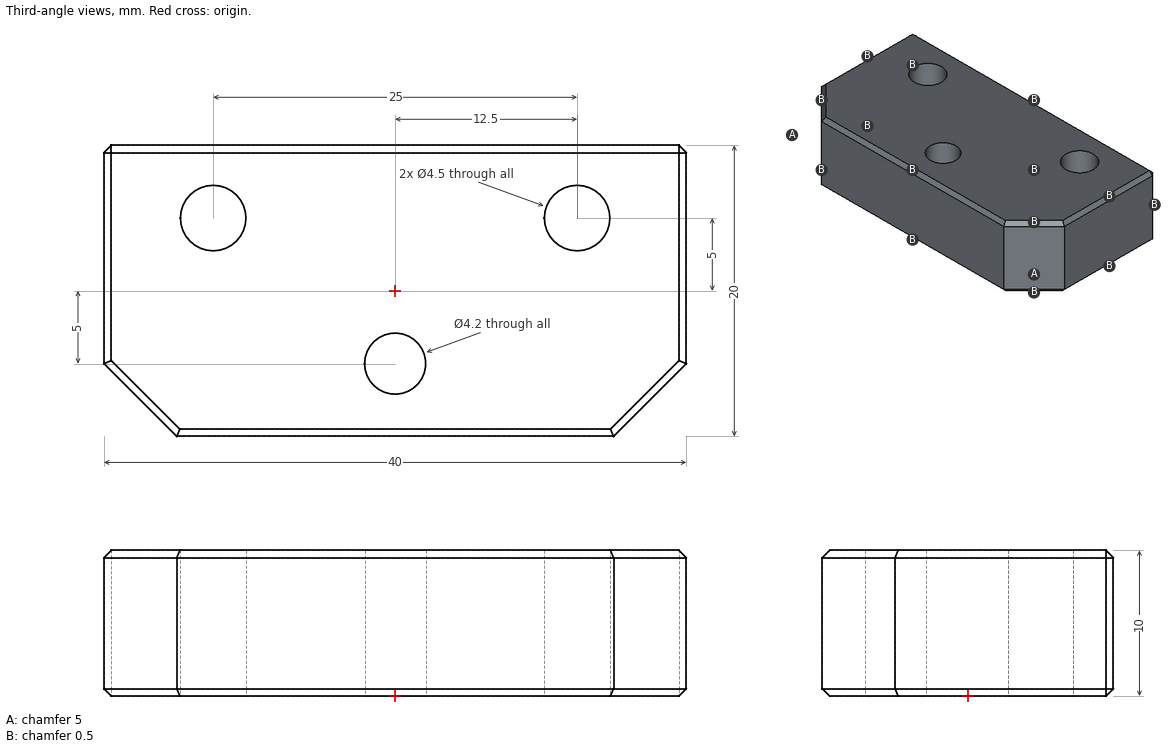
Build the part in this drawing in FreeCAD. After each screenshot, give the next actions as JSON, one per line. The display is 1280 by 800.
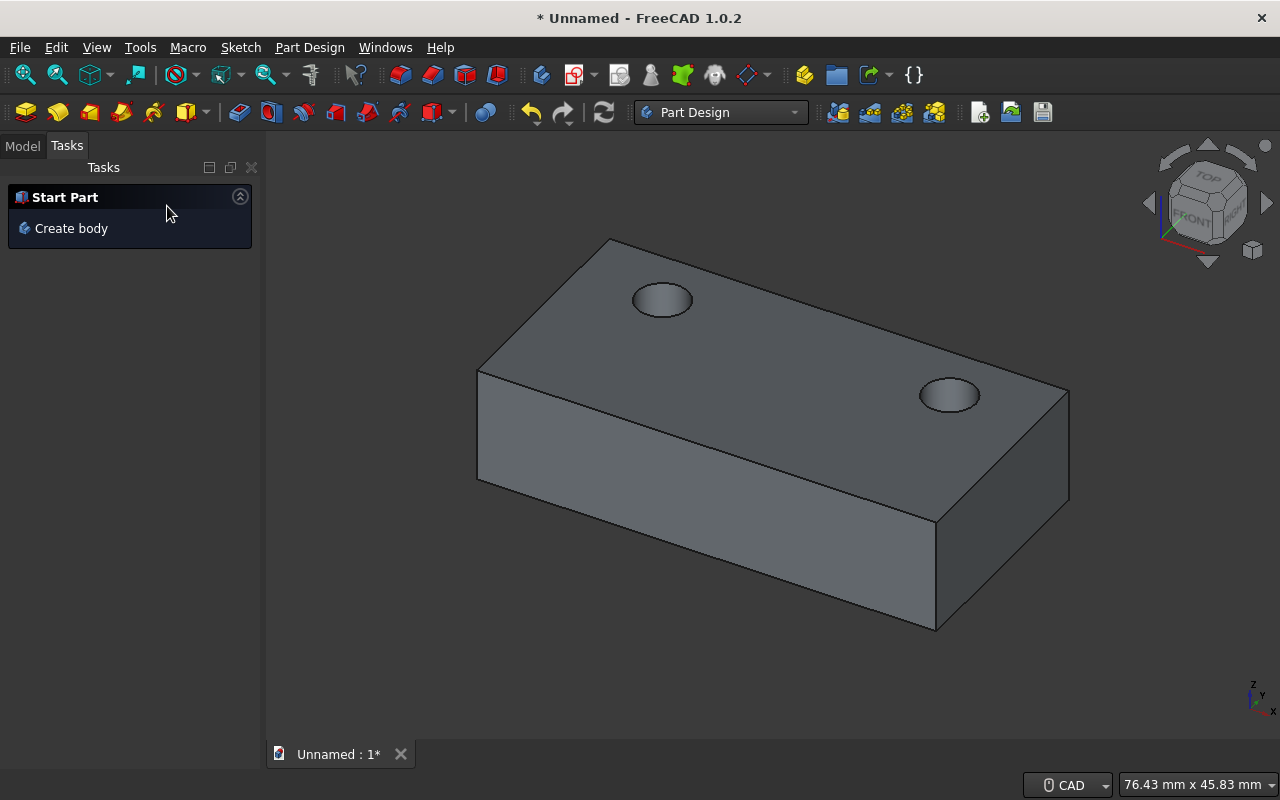
{"action": "left_click", "coordinate": [773, 380]}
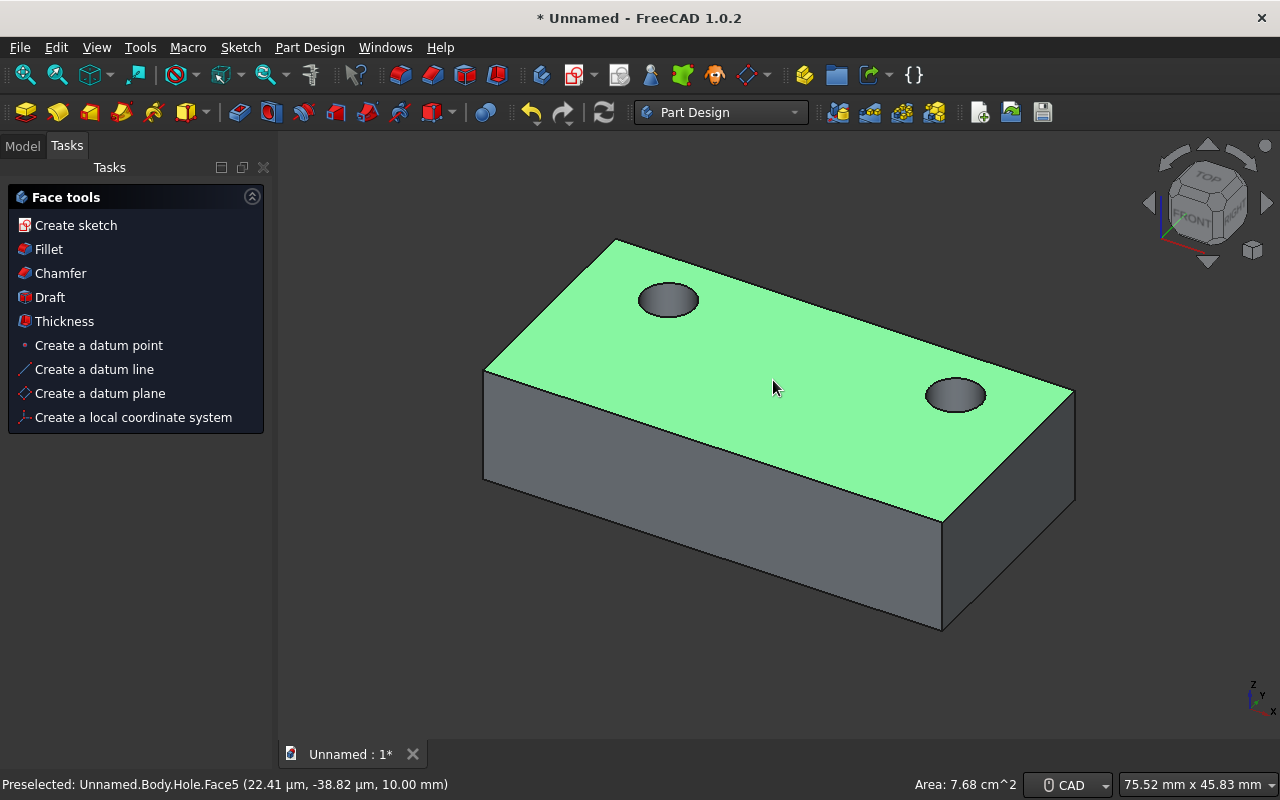
{"action": "left_click", "coordinate": [574, 76]}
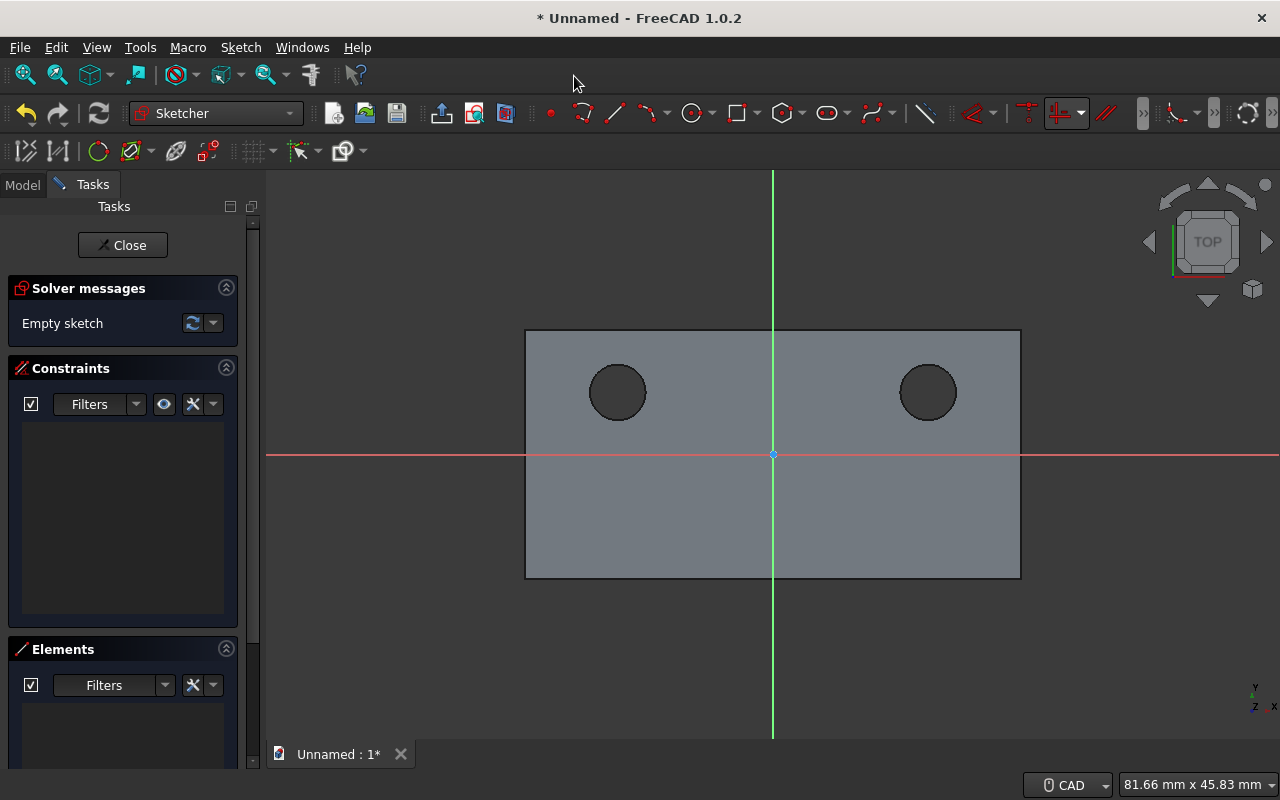
{"action": "scroll", "coordinate": [795, 513], "scroll_direction": "up", "scroll_amount": 7}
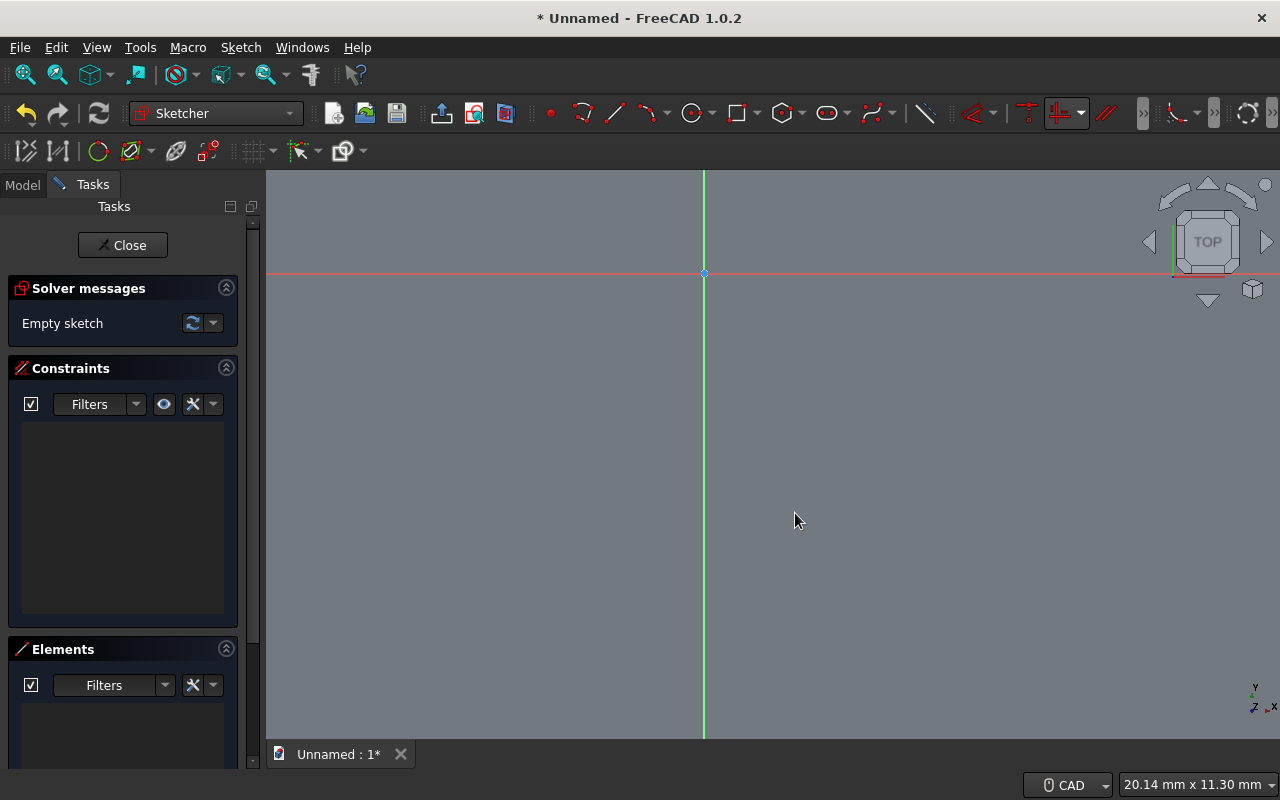
{"action": "left_click", "coordinate": [692, 114]}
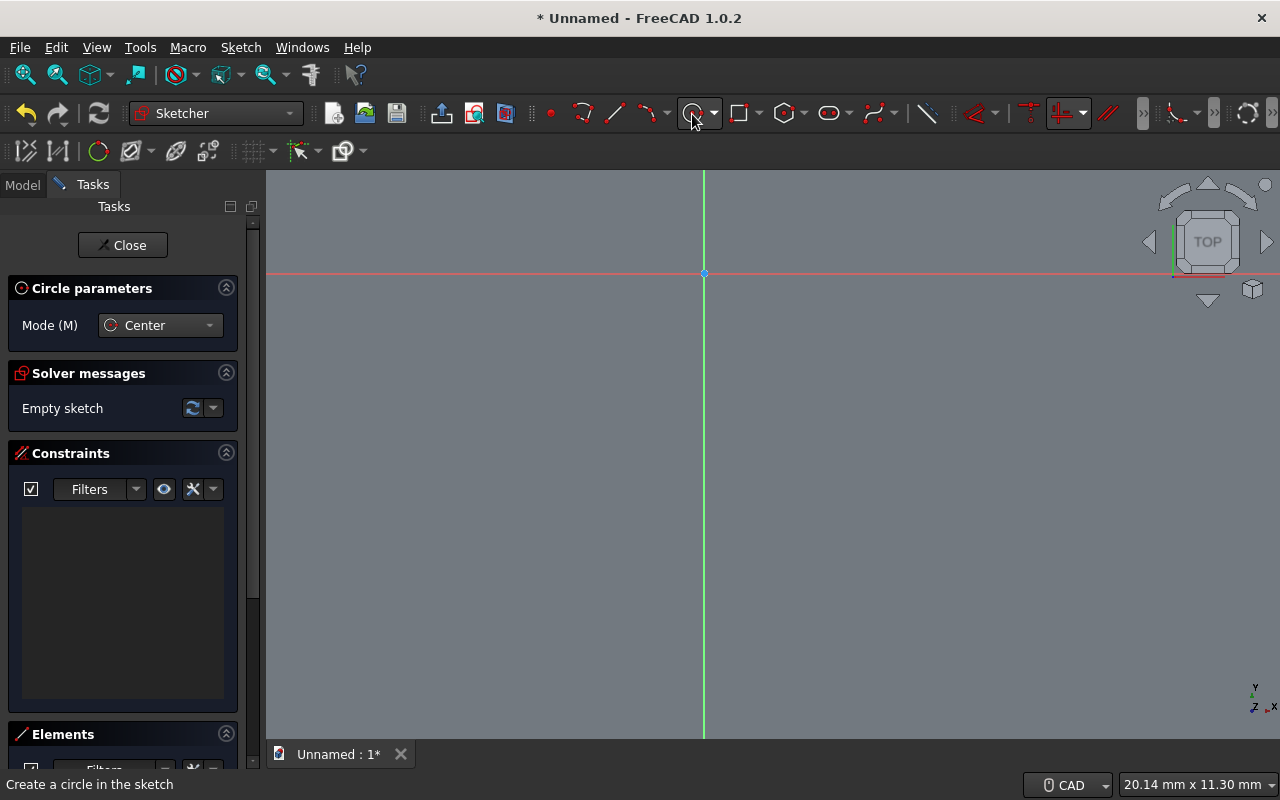
{"action": "left_click", "coordinate": [704, 526]}
{"action": "mouse_move", "coordinate": [779, 451]}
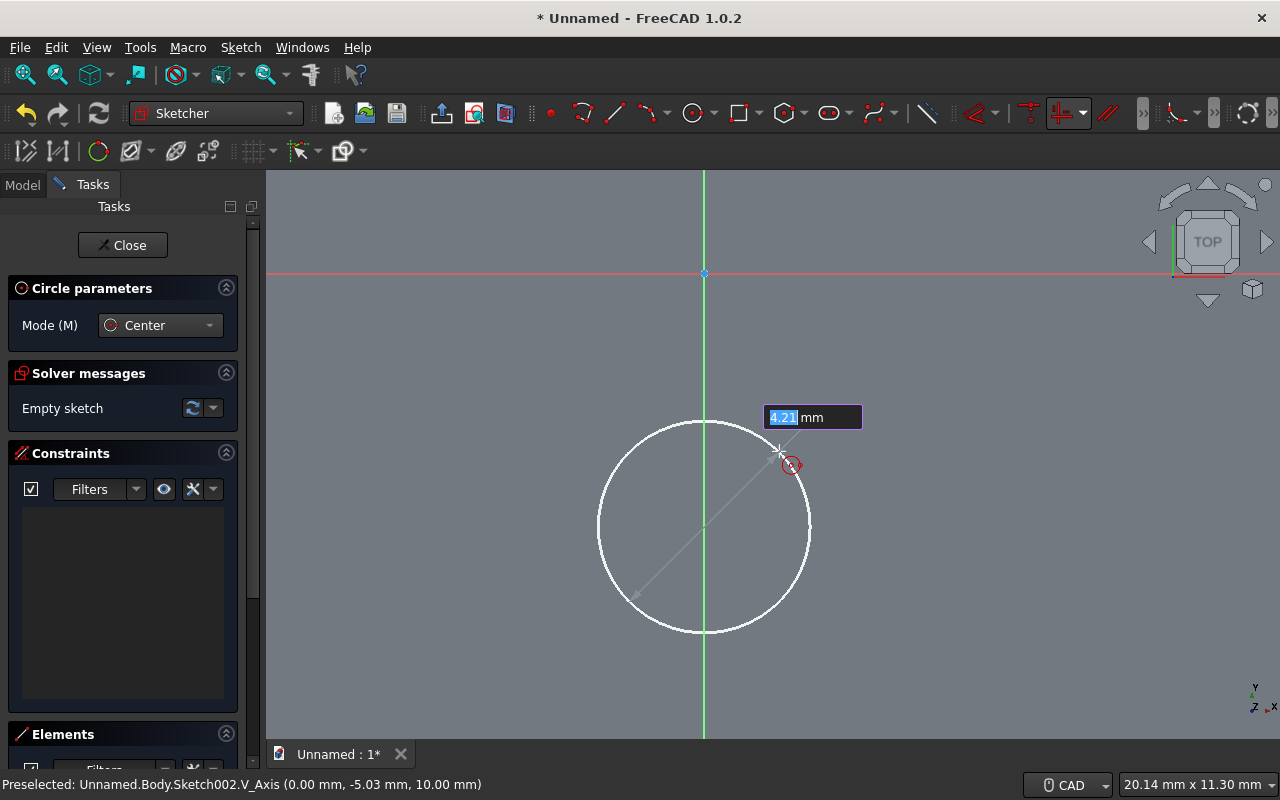
{"action": "type", "text": "4.2"}
{"action": "key", "text": "Return"}
{"action": "key", "text": "Escape"}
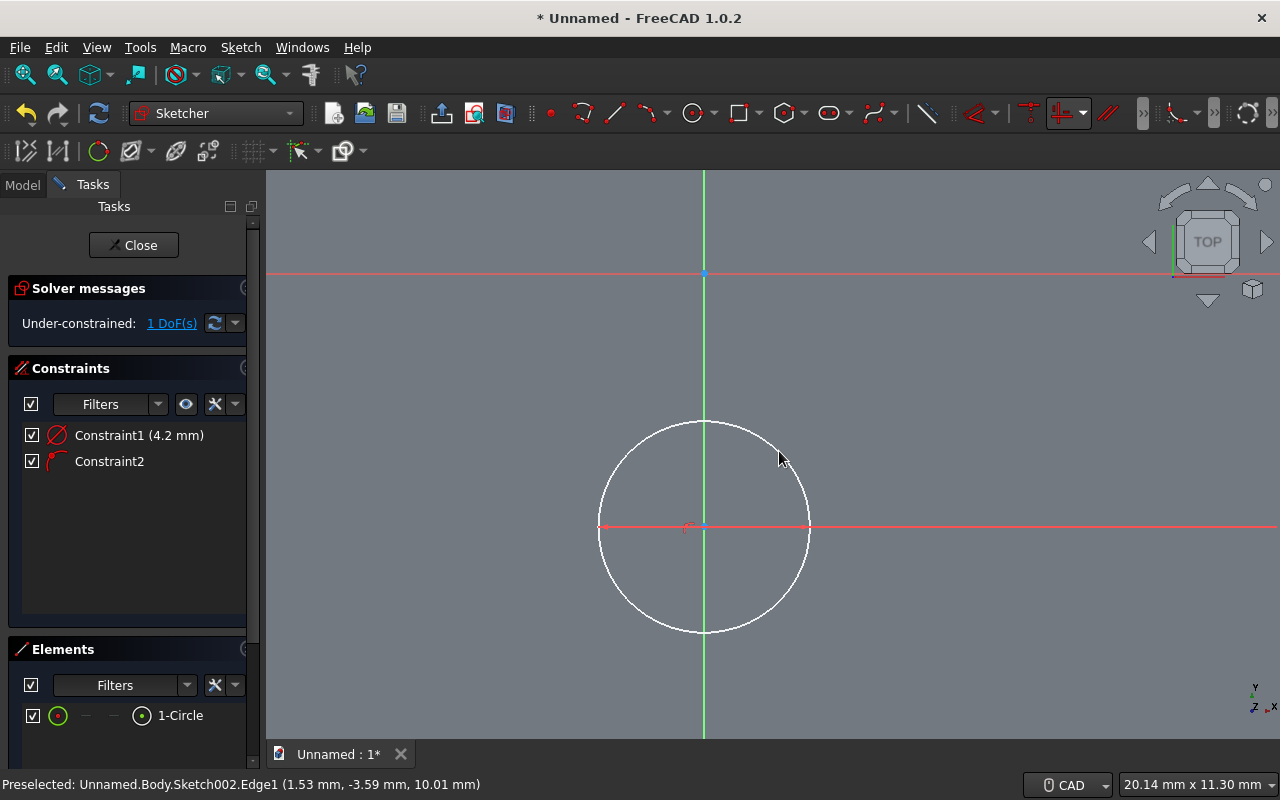
{"action": "left_click", "coordinate": [974, 114]}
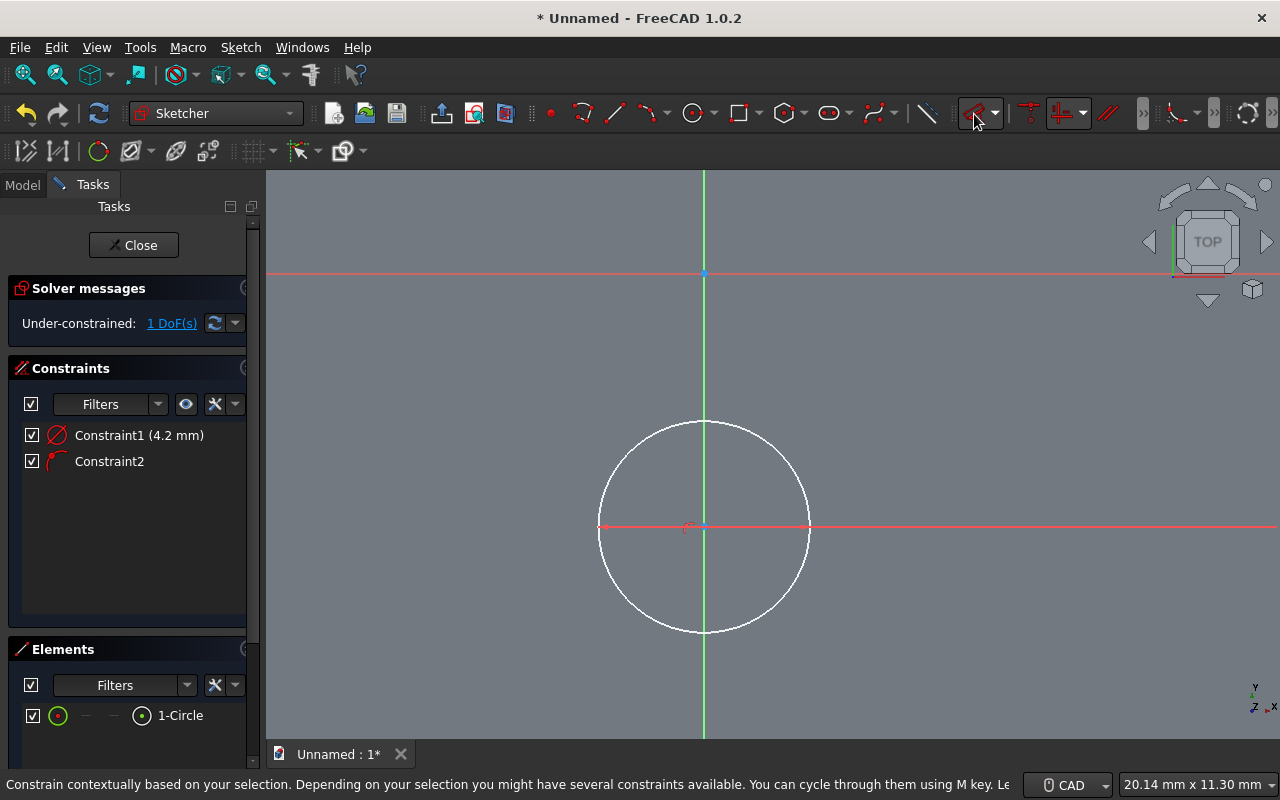
{"action": "left_click", "coordinate": [704, 527]}
{"action": "left_click", "coordinate": [738, 400]}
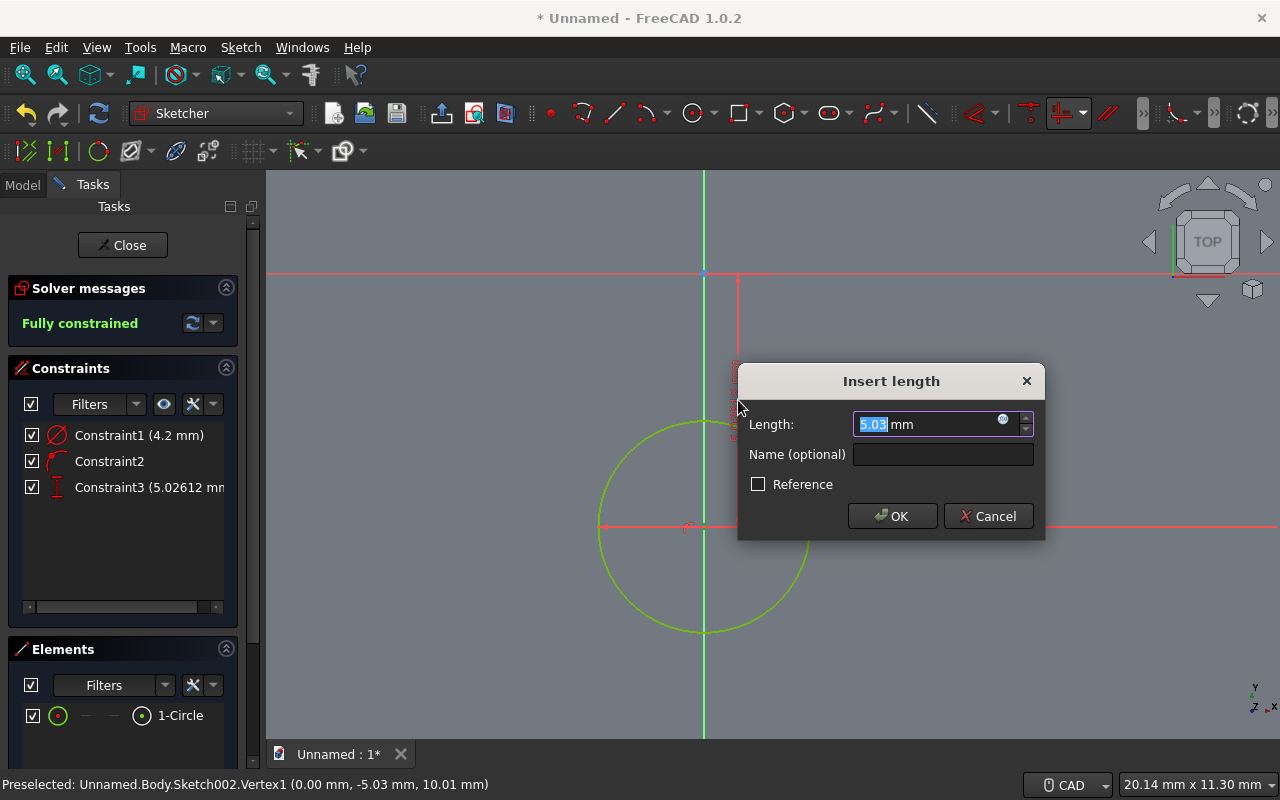
{"action": "type", "text": "5"}
{"action": "key", "text": "Return"}
{"action": "key", "text": "Escape"}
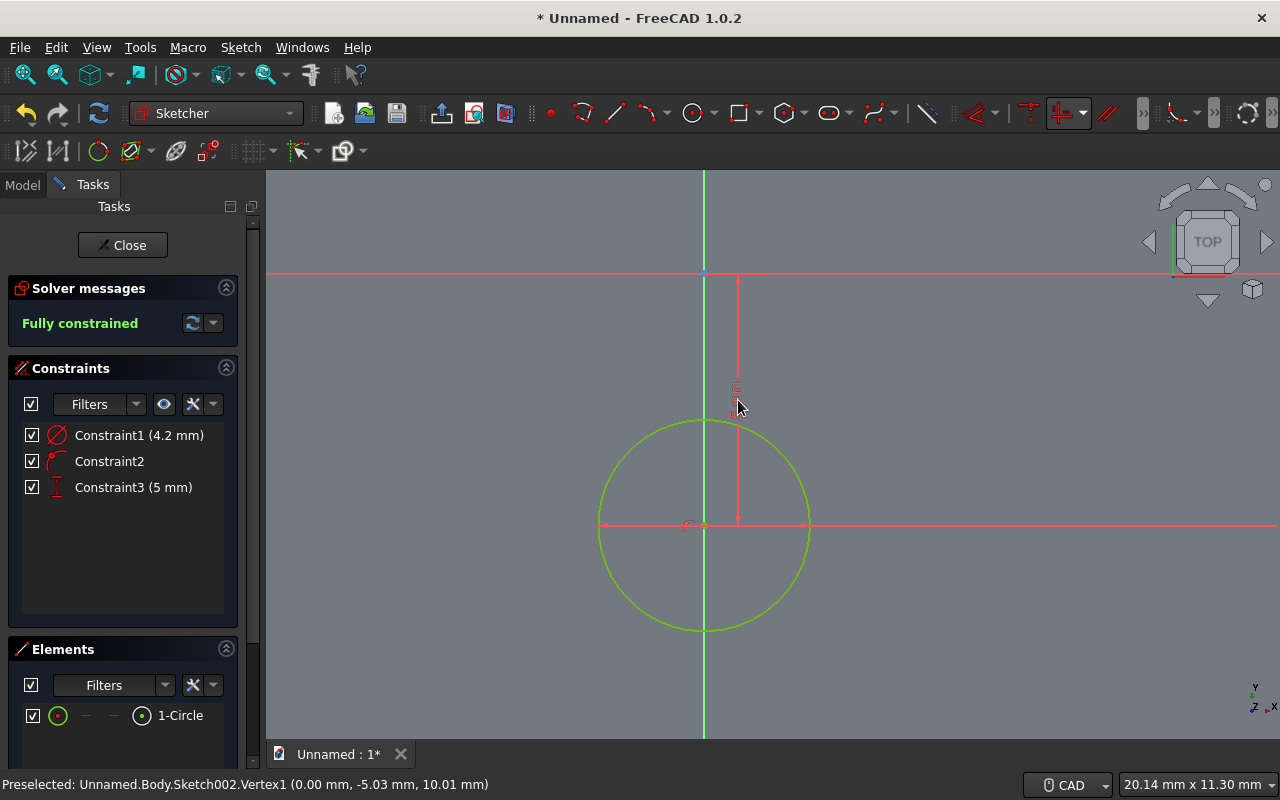
{"action": "left_click", "coordinate": [123, 245]}